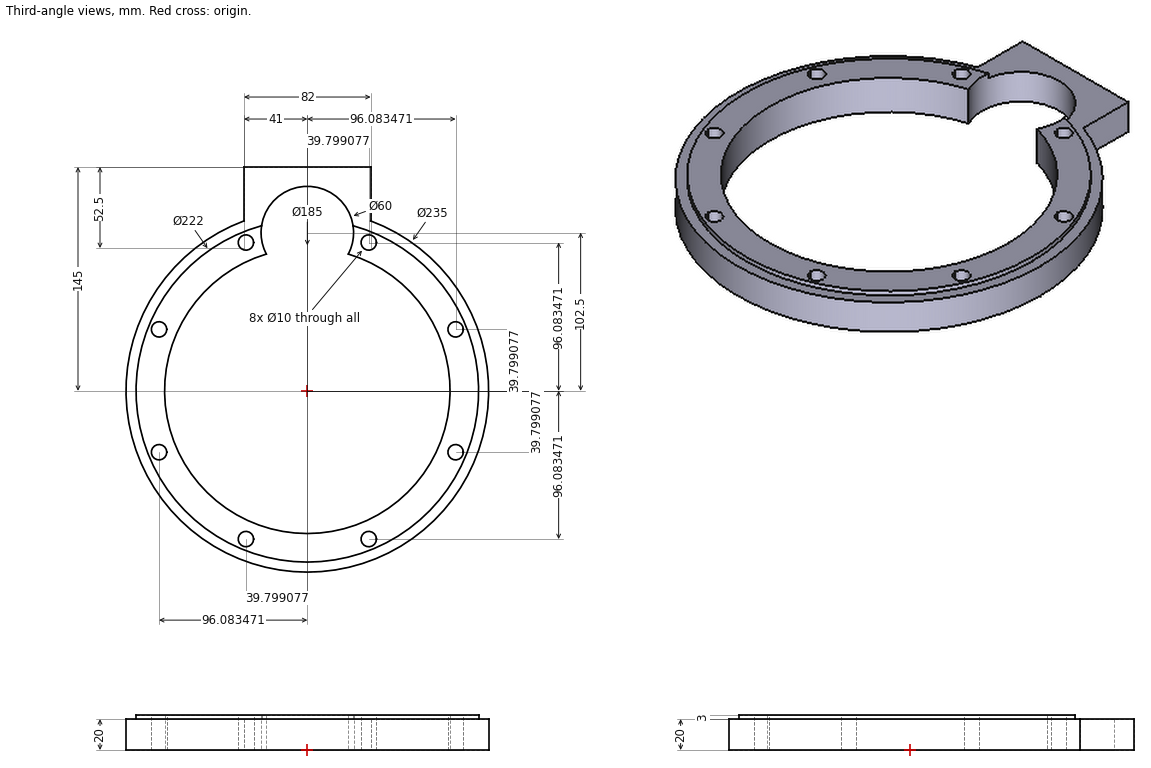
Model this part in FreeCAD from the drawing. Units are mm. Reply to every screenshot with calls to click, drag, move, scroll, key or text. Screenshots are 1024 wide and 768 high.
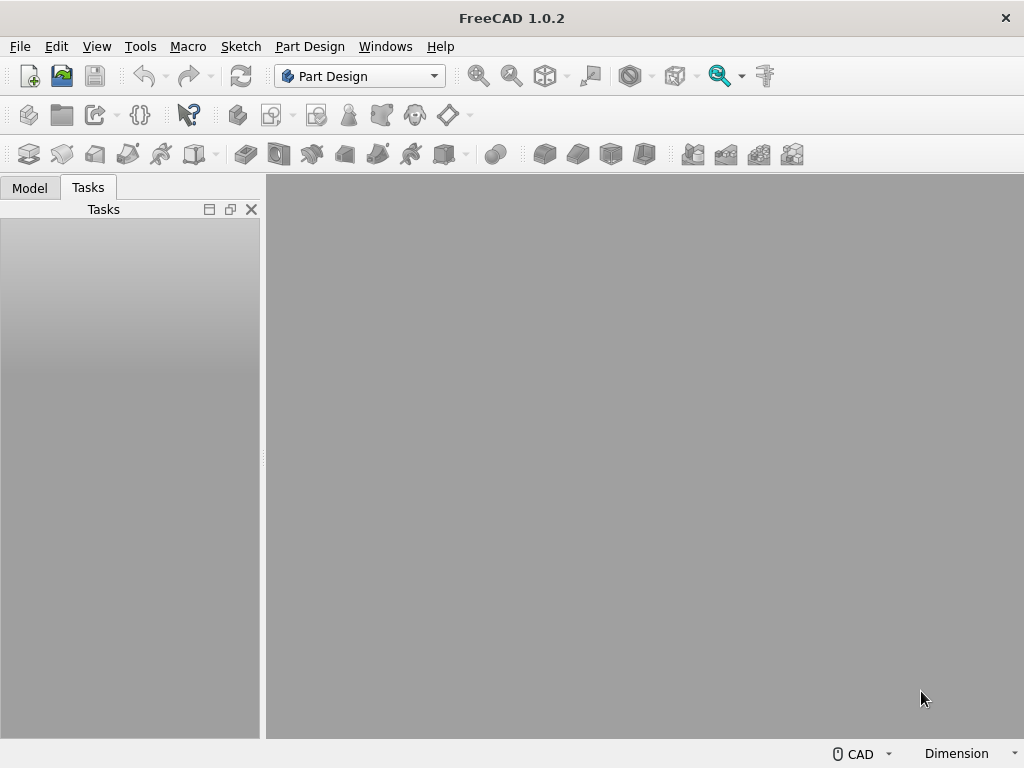
click(29, 76)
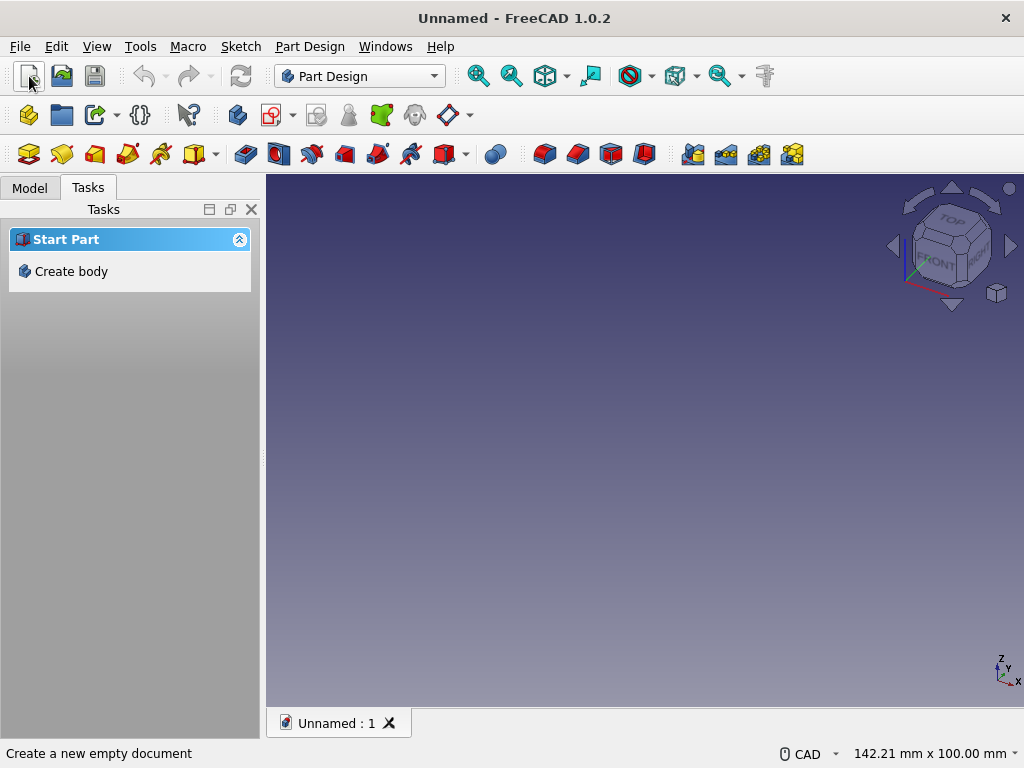
click(270, 116)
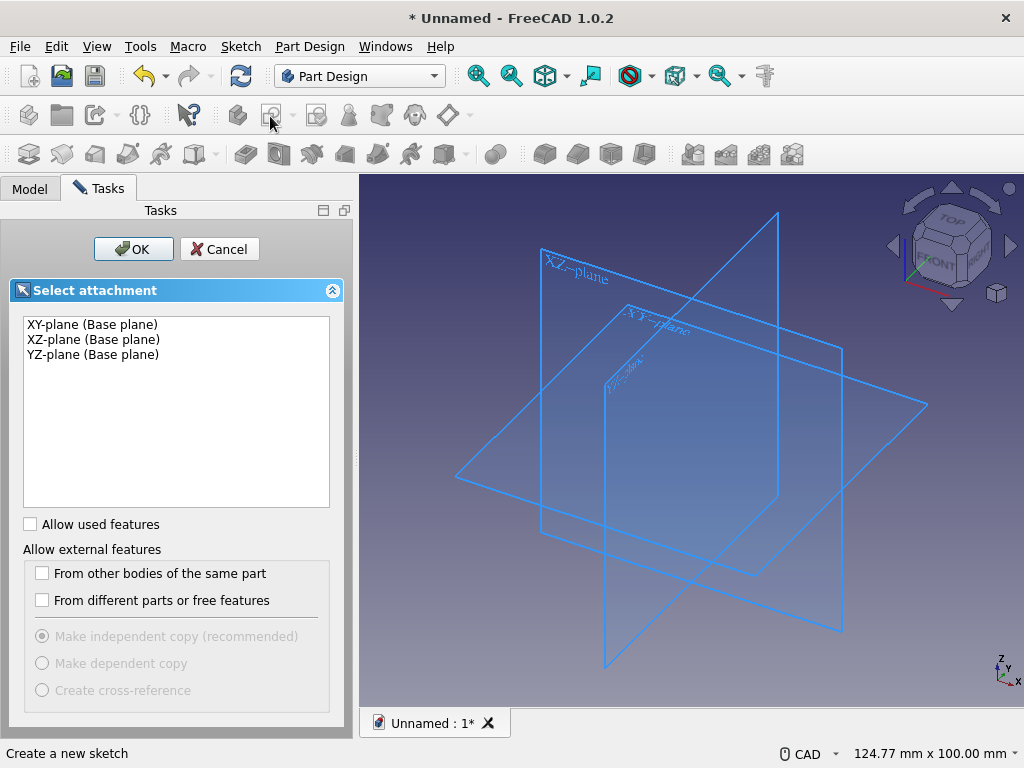
click(84, 324)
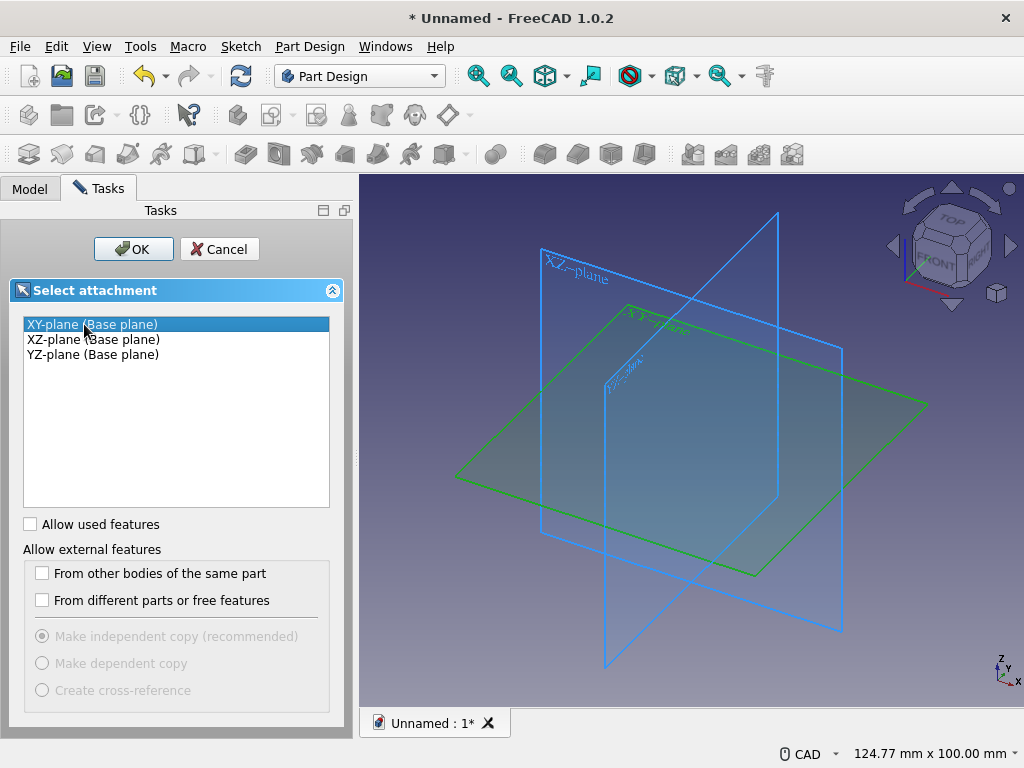
click(134, 249)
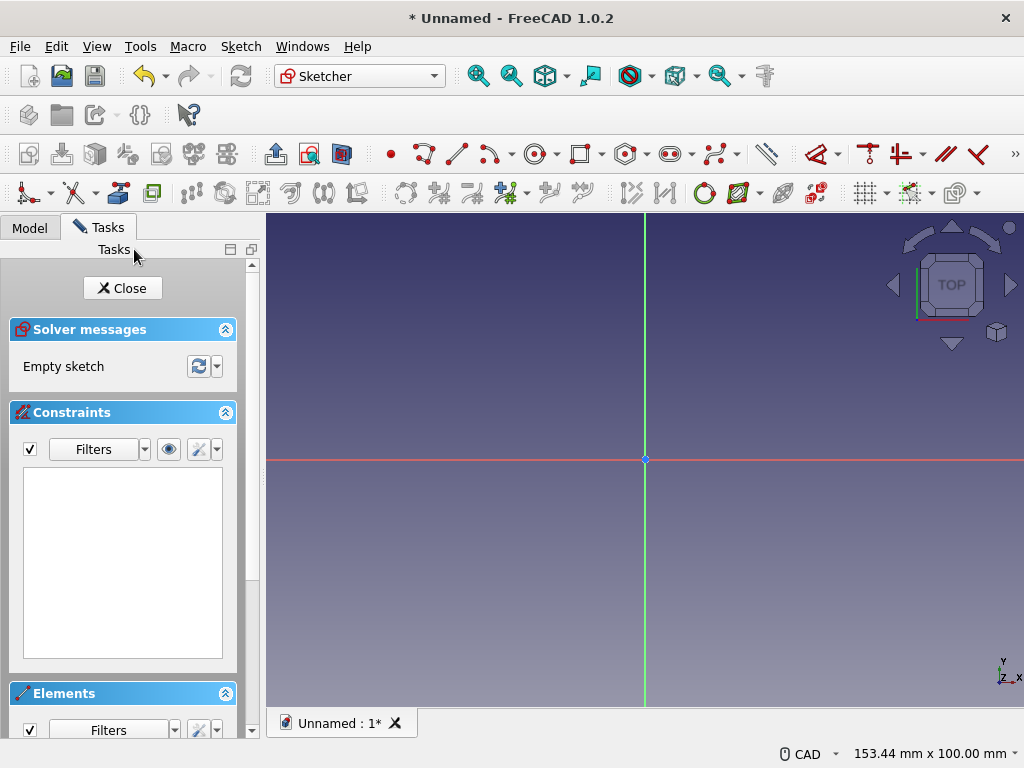
scroll(554, 460, down, 7)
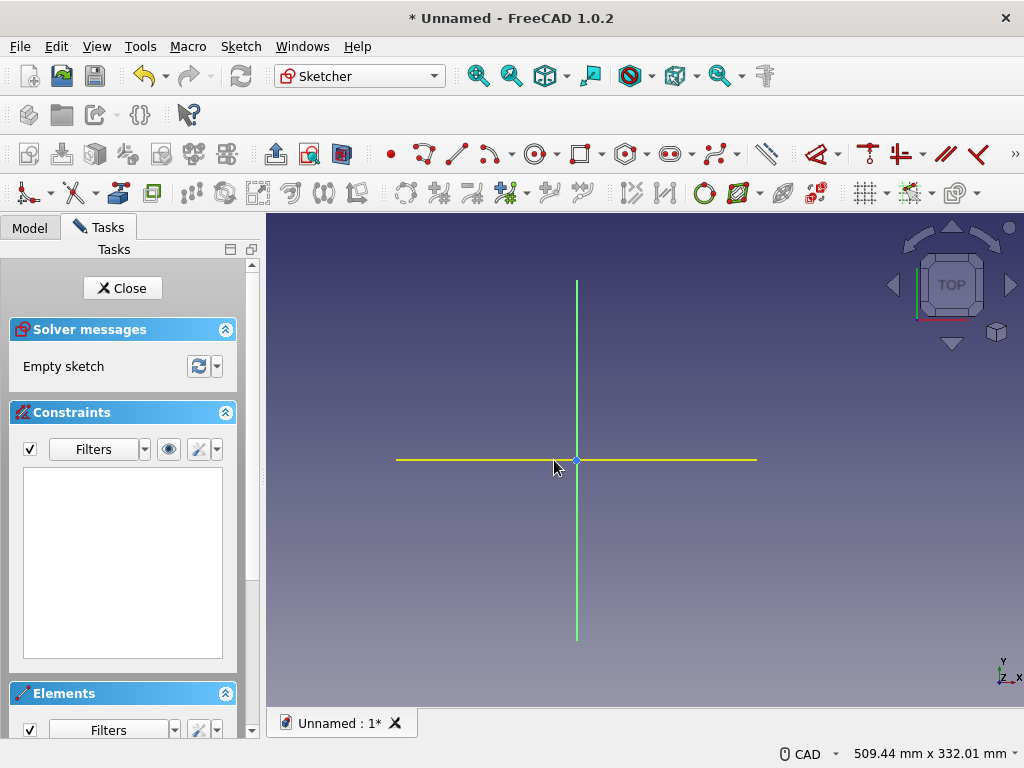
click(534, 154)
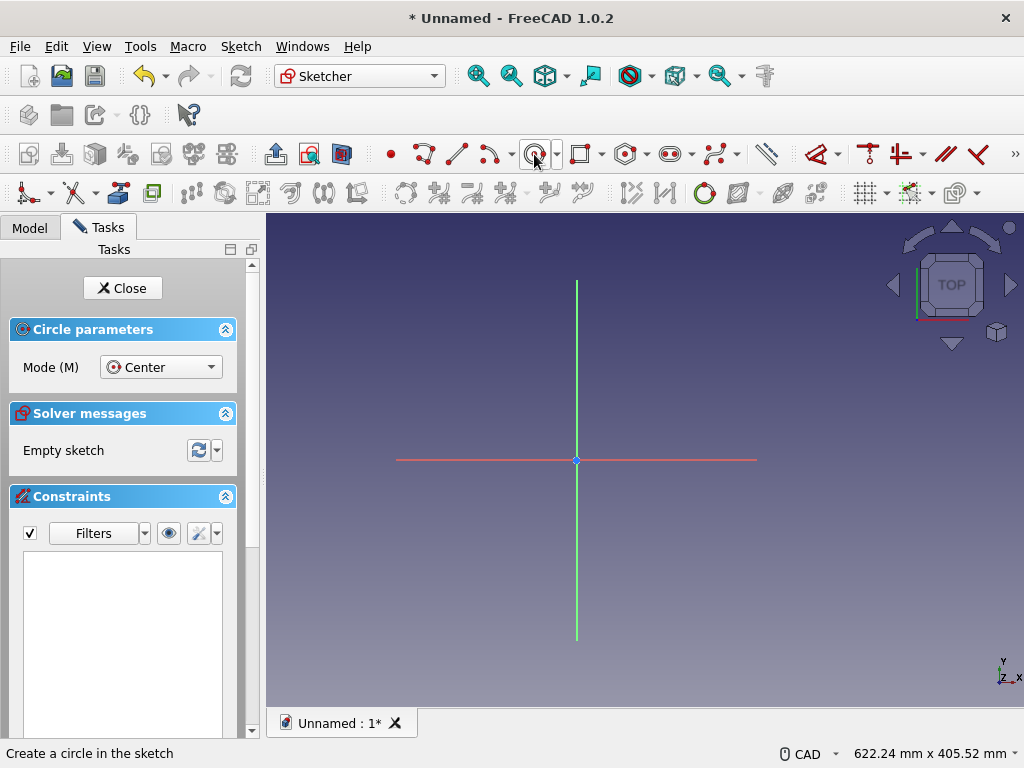
click(577, 460)
click(678, 359)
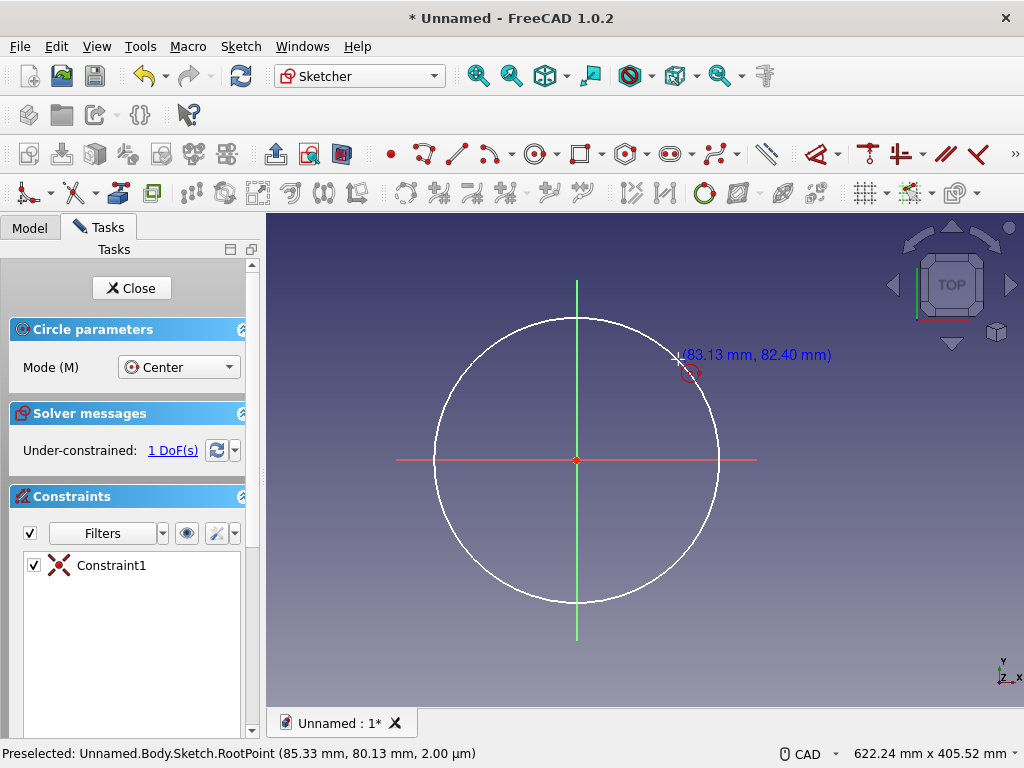
click(577, 460)
click(656, 381)
key(Escape)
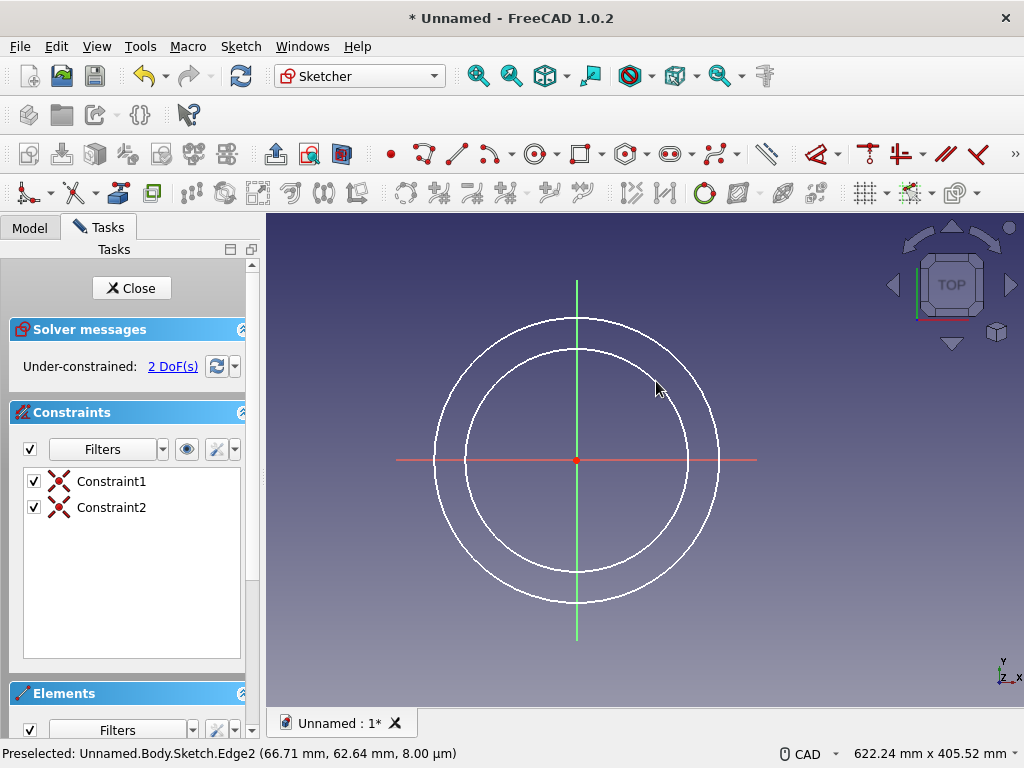
click(677, 359)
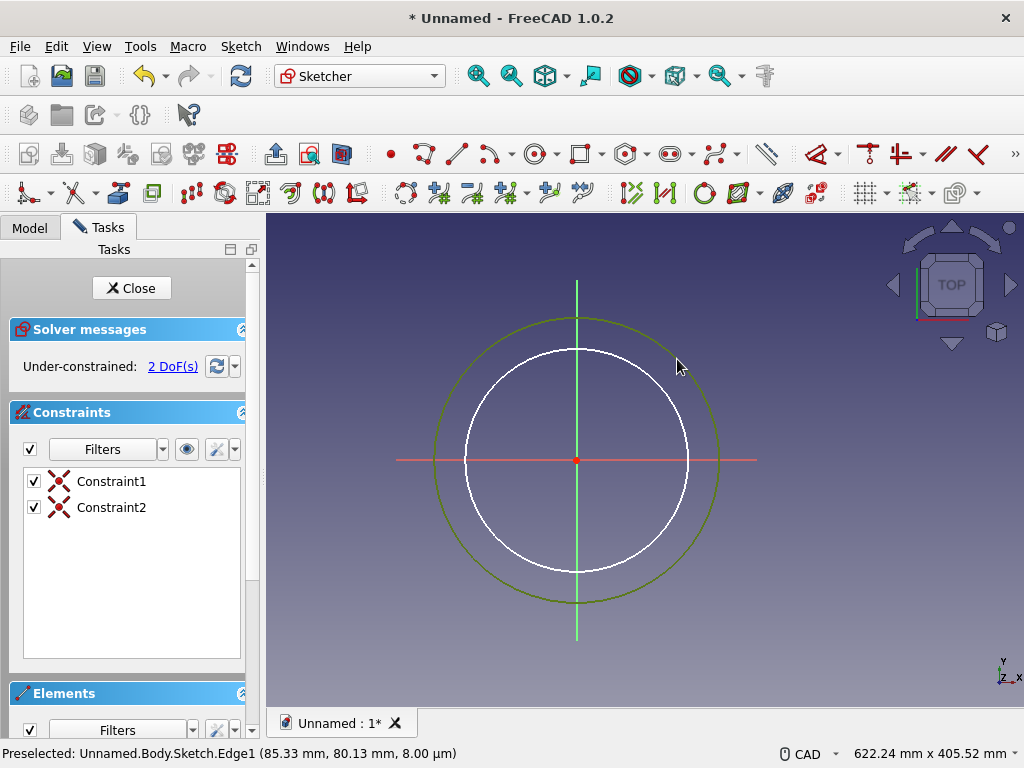
key(k)
key(o)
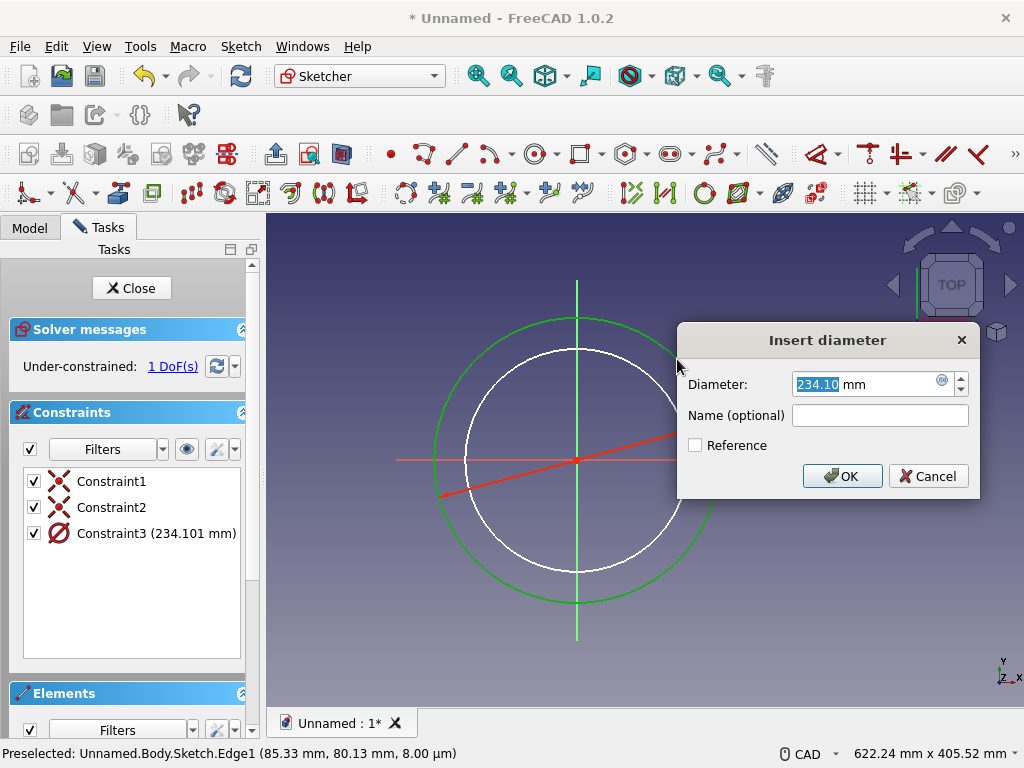
text(235)
key(Return)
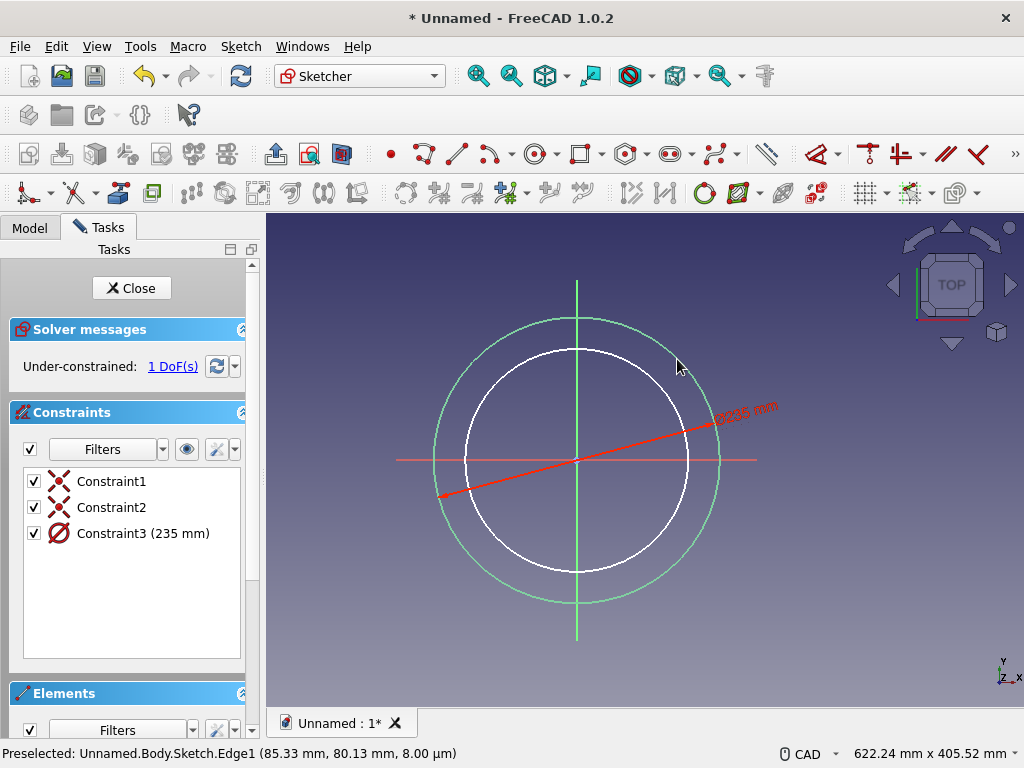
click(655, 381)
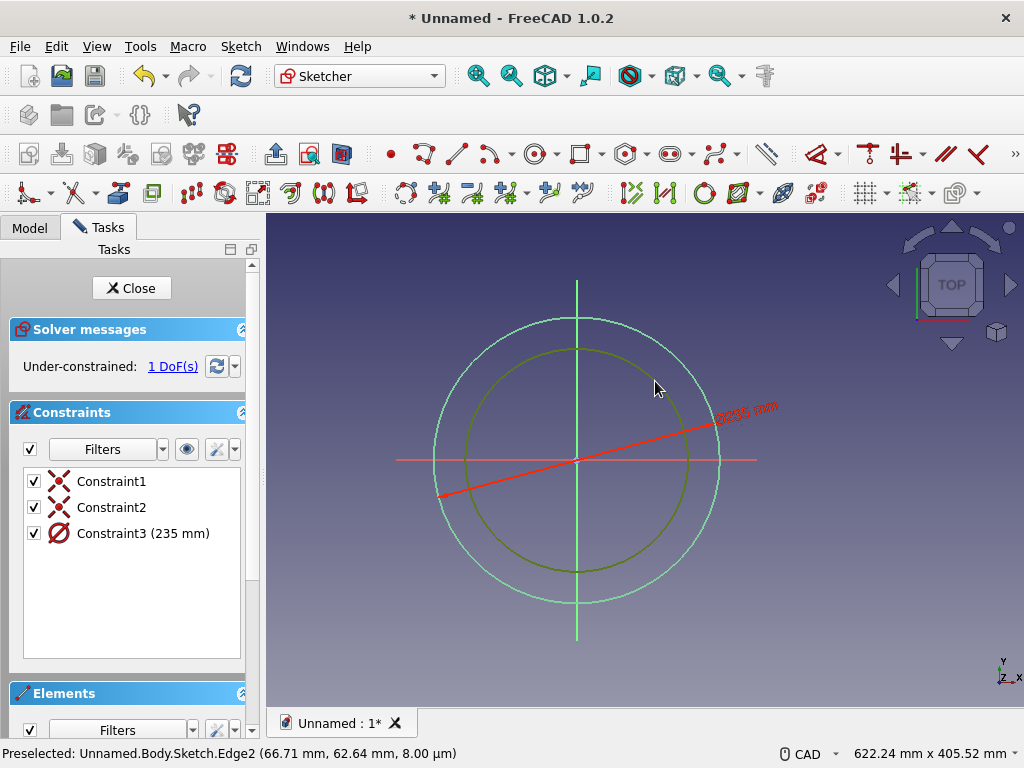
key(k)
key(o)